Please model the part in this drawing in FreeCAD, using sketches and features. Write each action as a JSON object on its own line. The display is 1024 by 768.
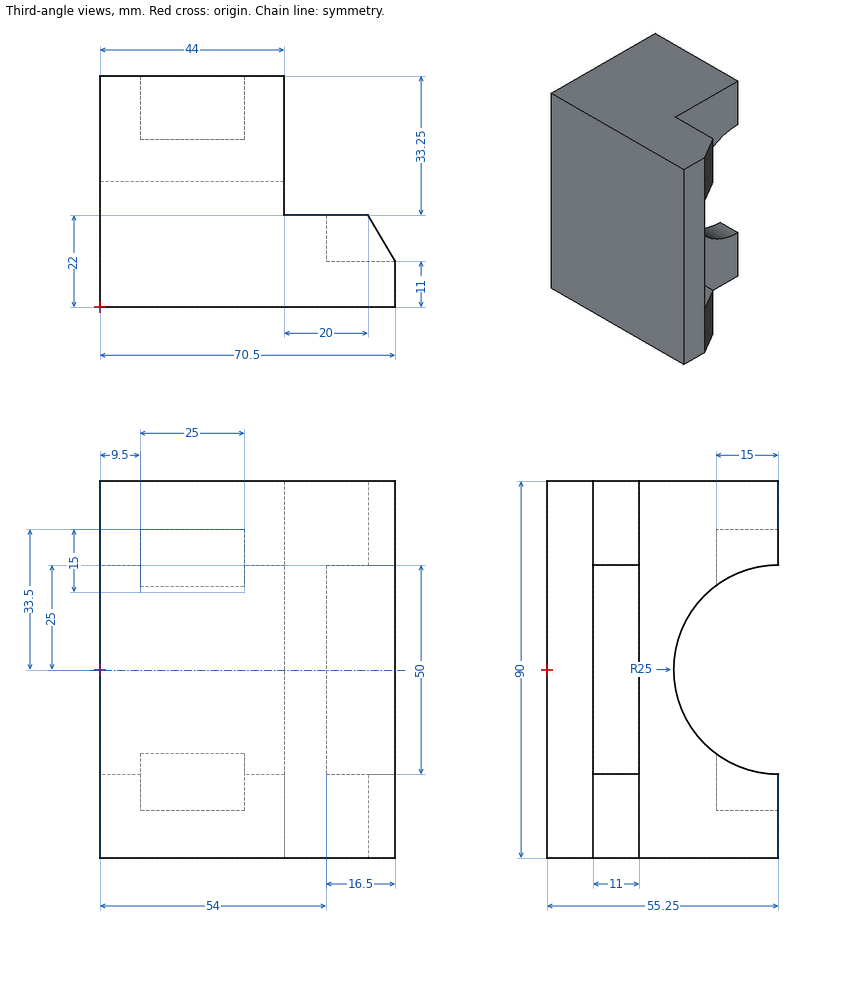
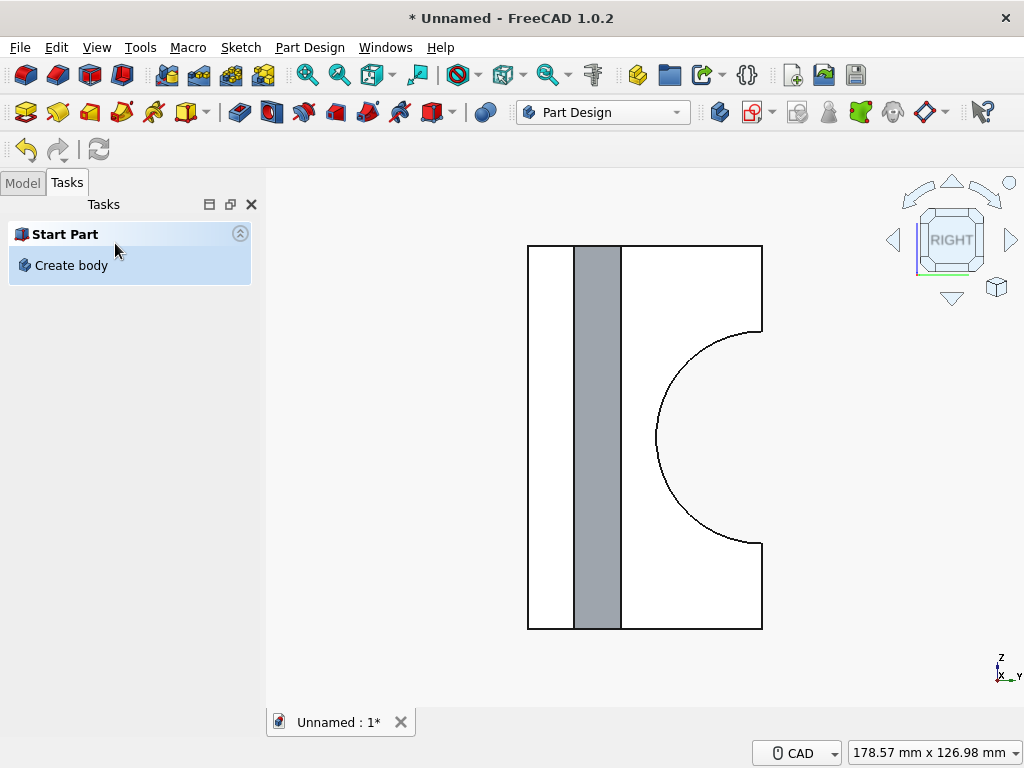
{"action": "key", "text": "4"}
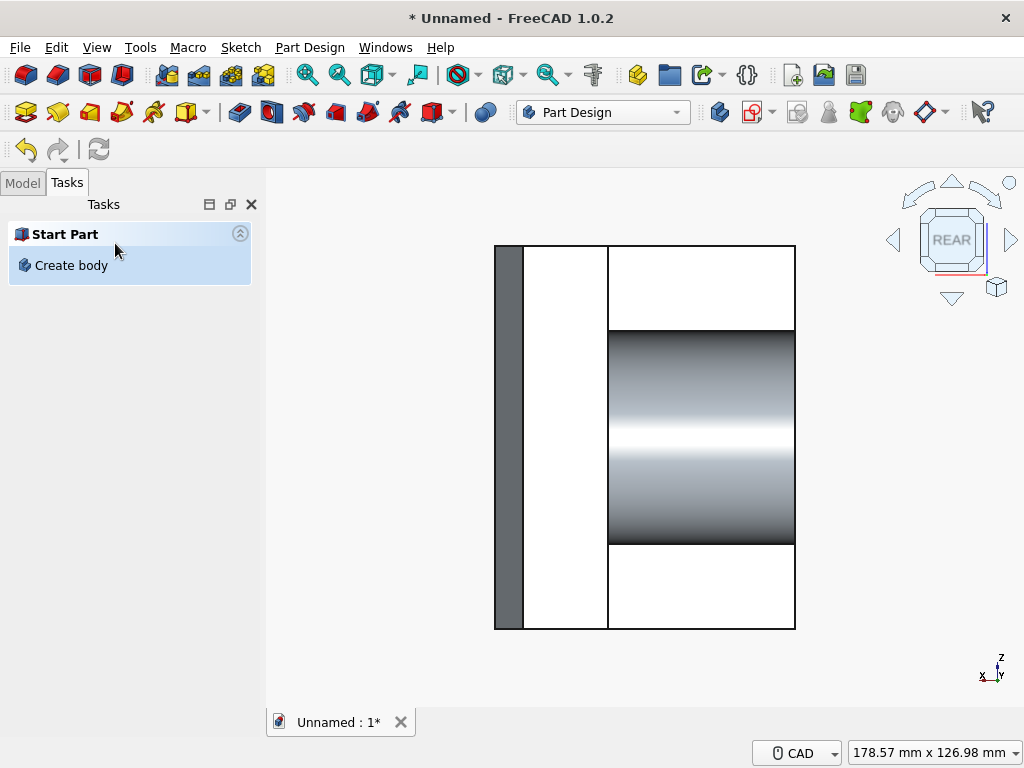
{"action": "left_click", "coordinate": [565, 327]}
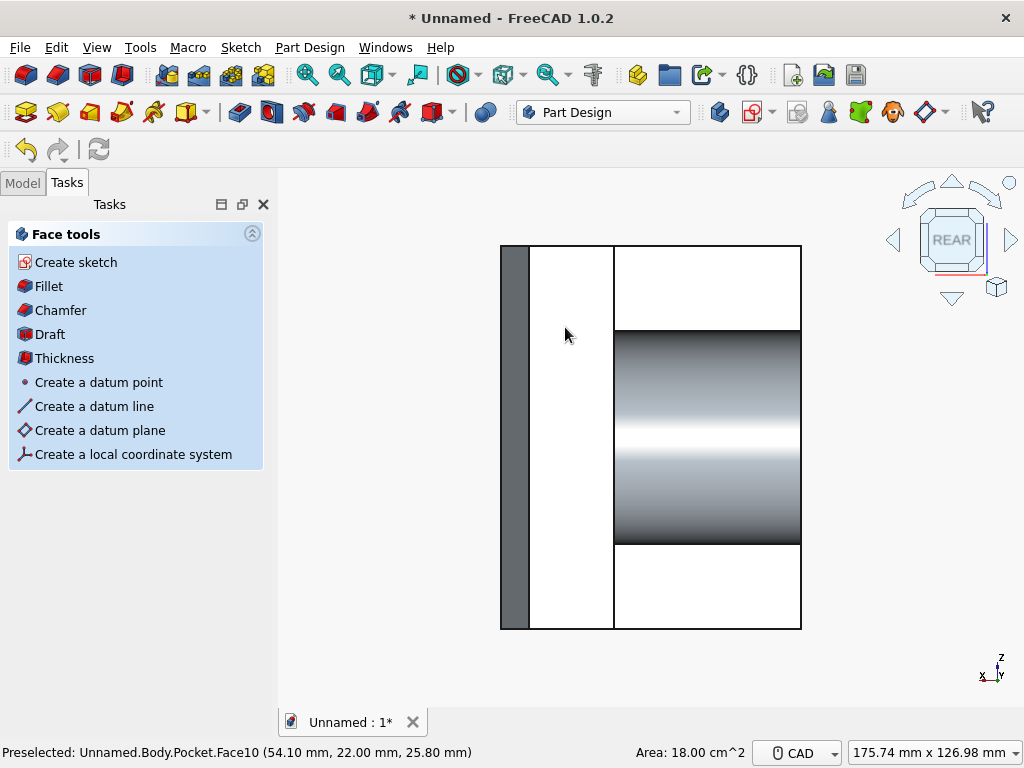
{"action": "left_click", "coordinate": [752, 112]}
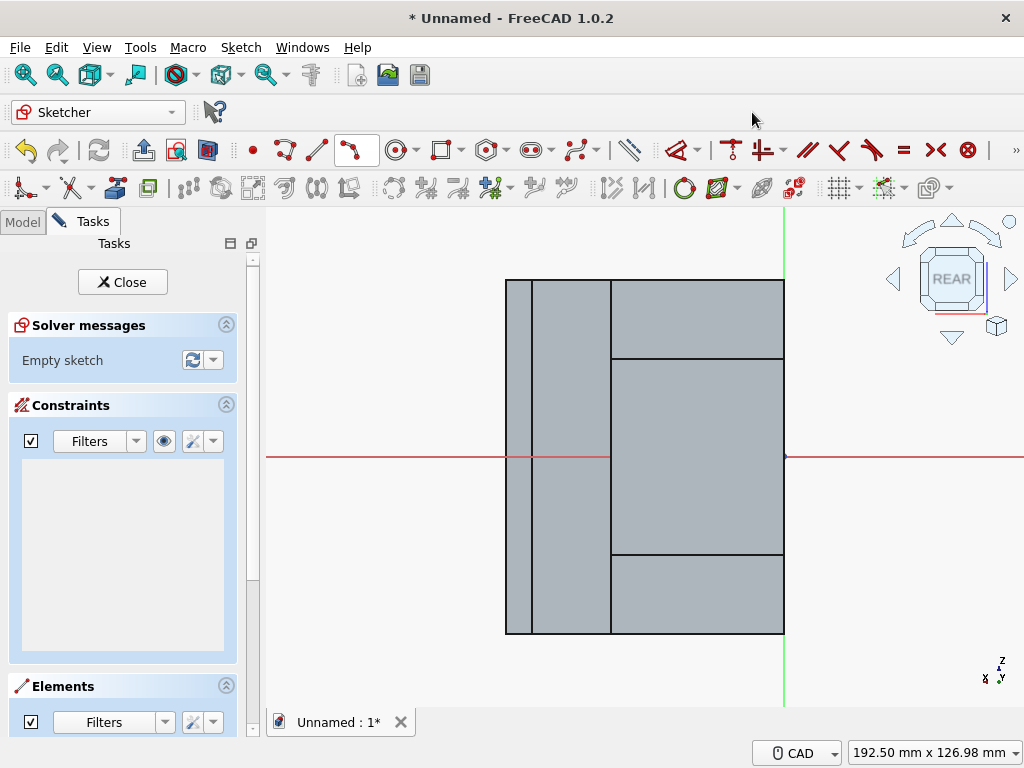
{"action": "left_click", "coordinate": [208, 150]}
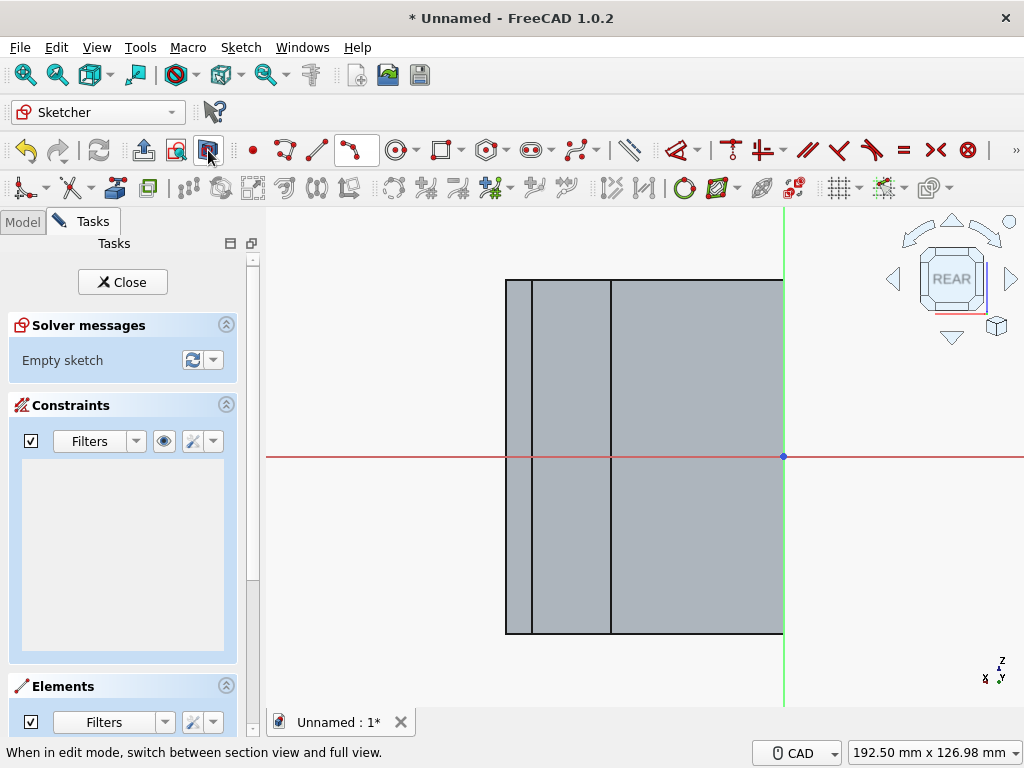
{"action": "scroll", "coordinate": [784, 457], "scroll_direction": "up", "scroll_amount": 2}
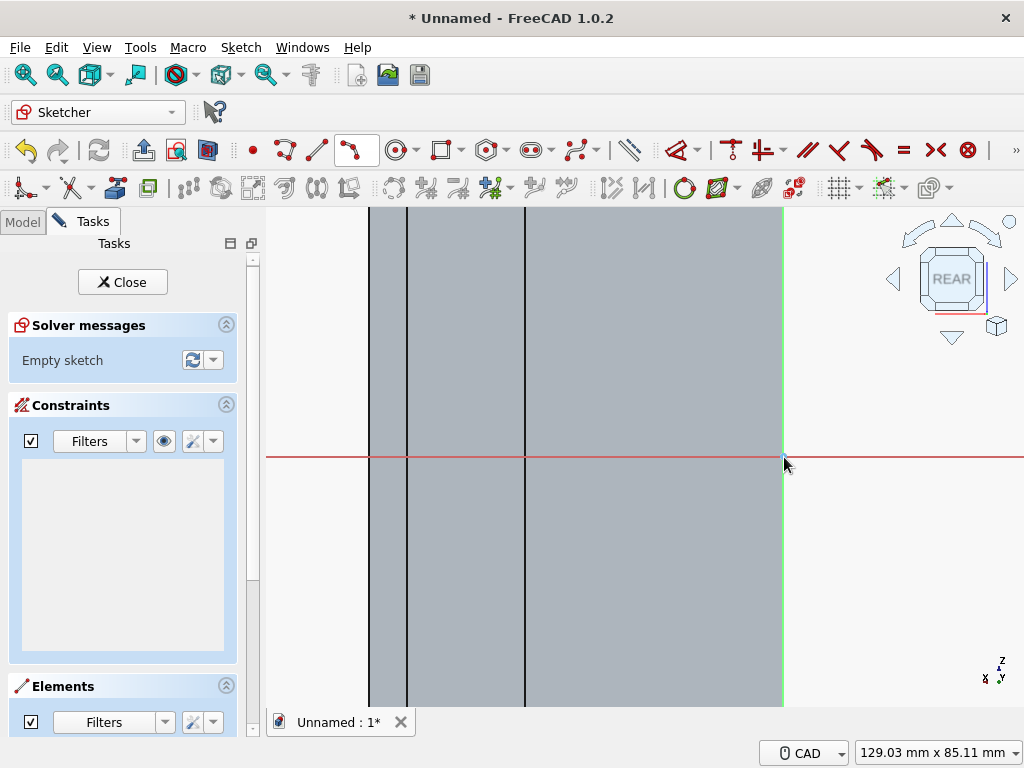
{"action": "left_click", "coordinate": [442, 150]}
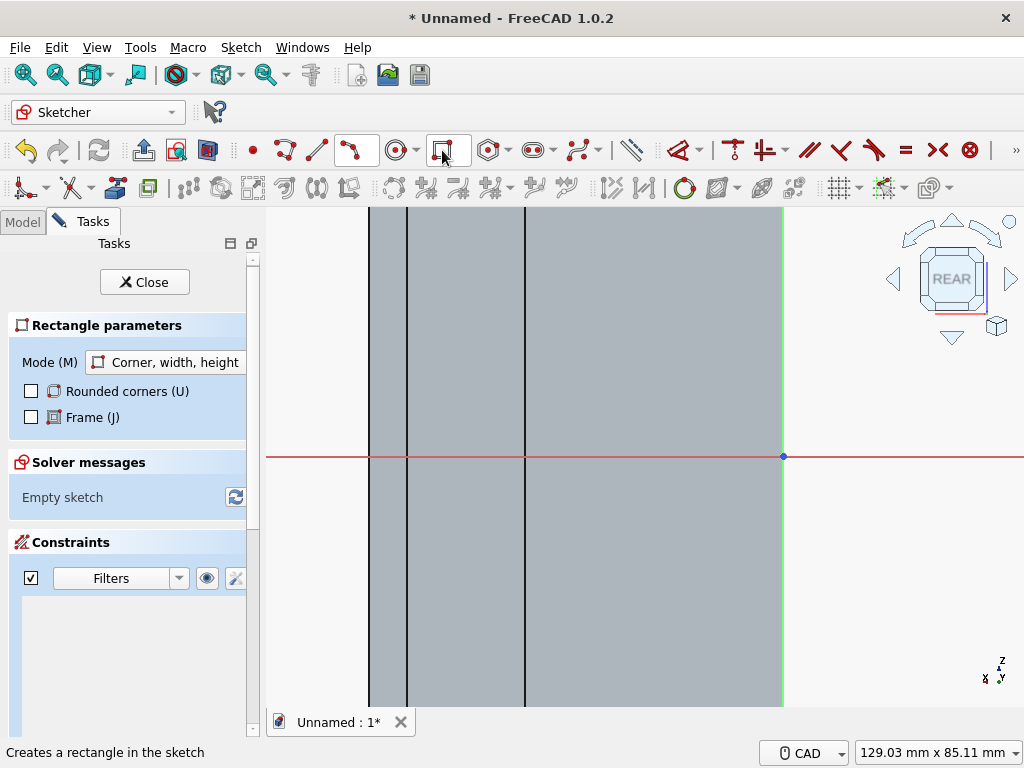
{"action": "left_click", "coordinate": [369, 310]}
{"action": "left_click", "coordinate": [466, 604]}
{"action": "key", "text": "Escape"}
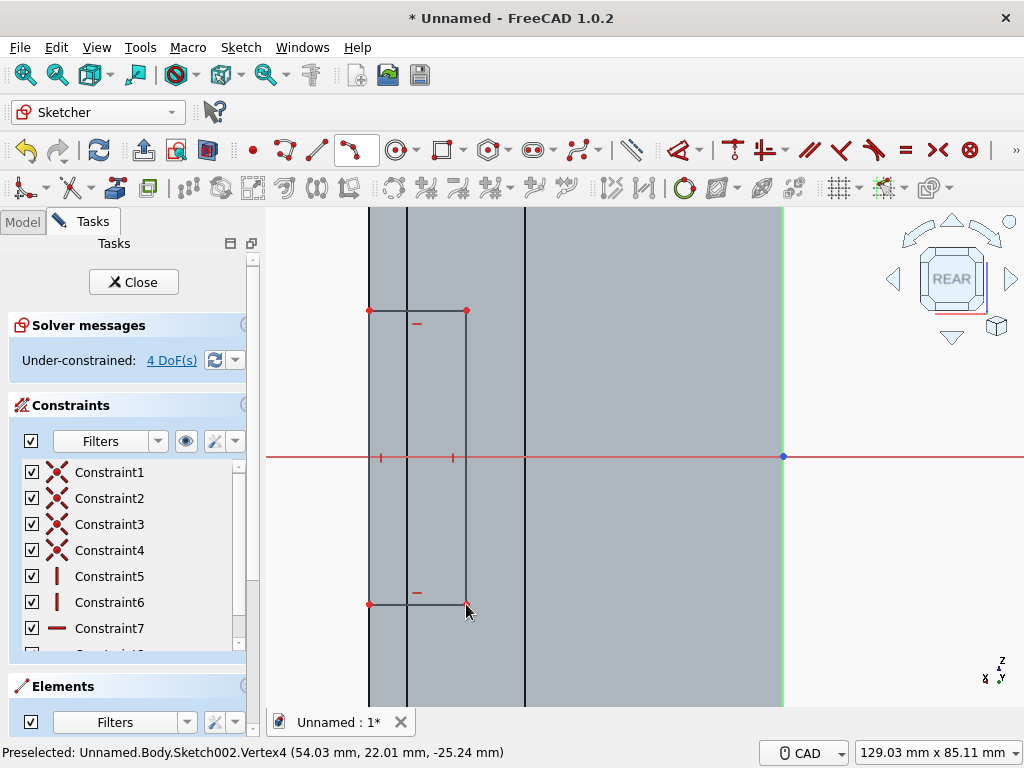
{"action": "left_click", "coordinate": [678, 150]}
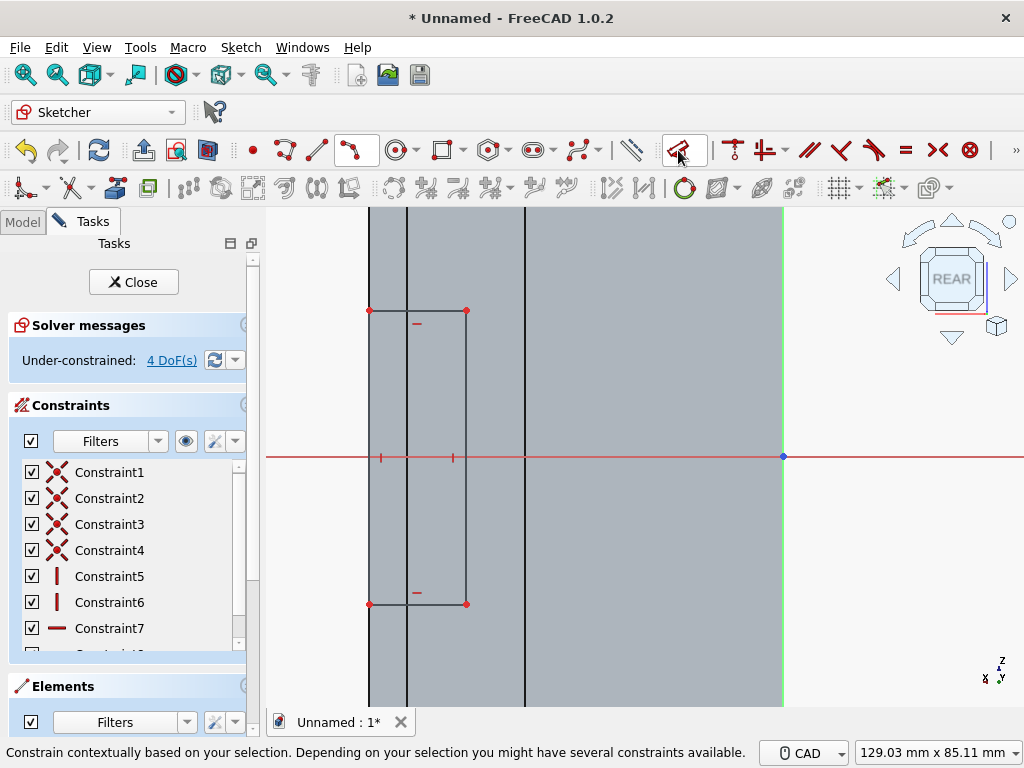
{"action": "left_click", "coordinate": [369, 399]}
{"action": "left_click", "coordinate": [335, 390]}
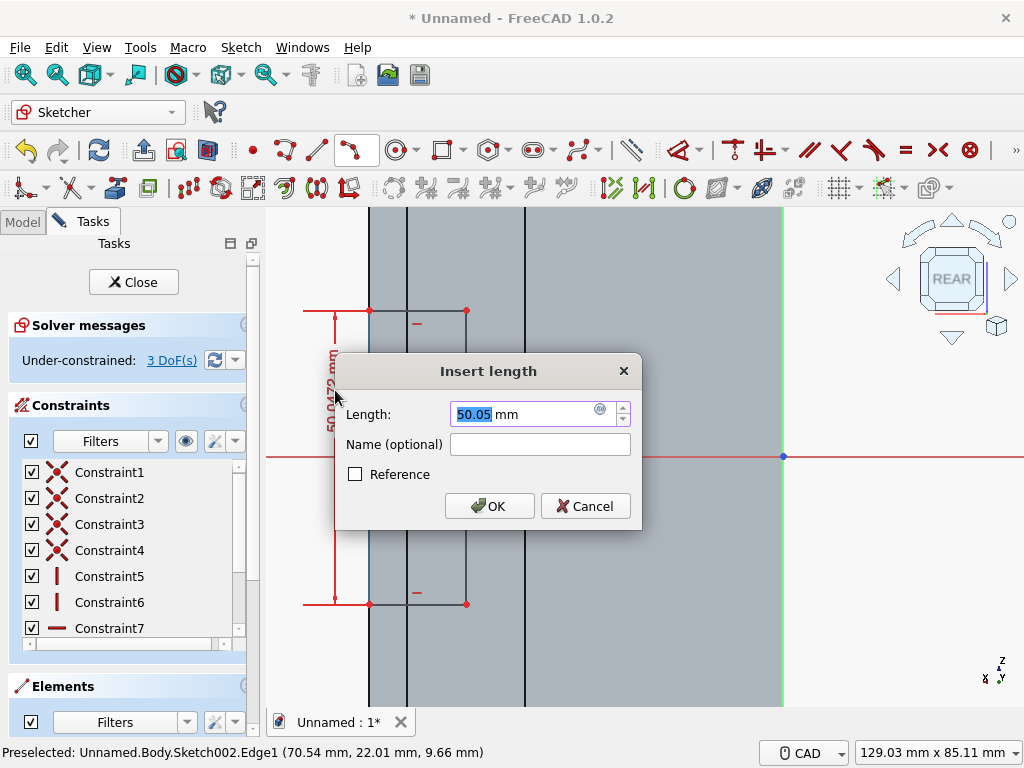
{"action": "type", "text": "50"}
{"action": "key", "text": "Return"}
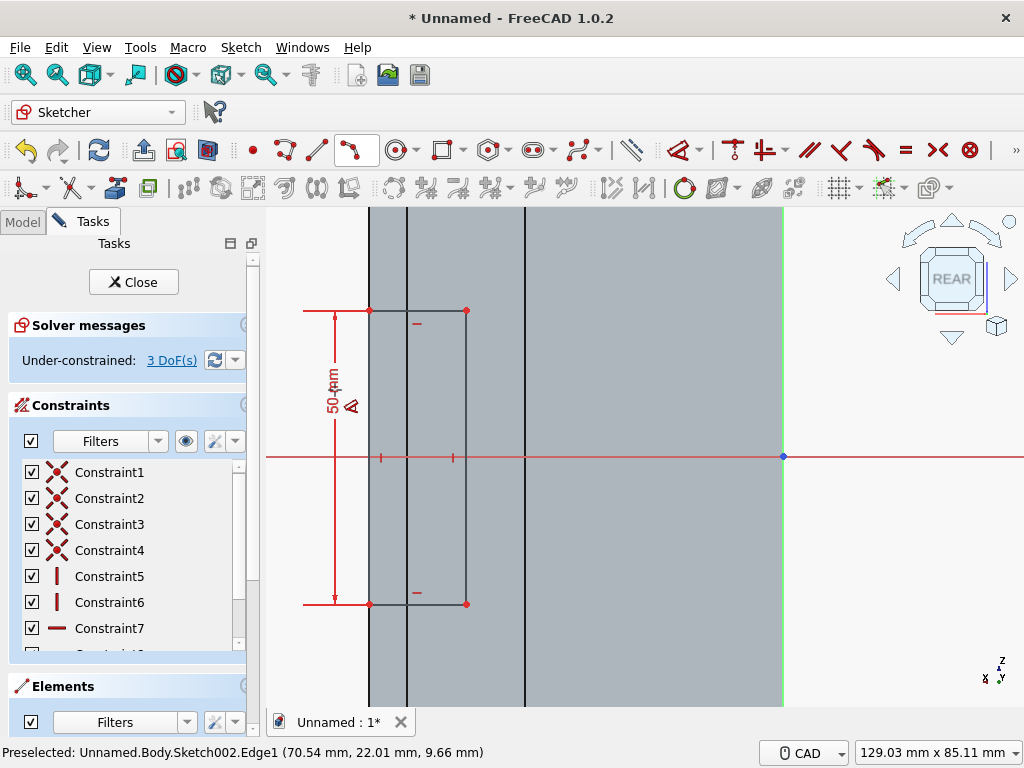
{"action": "left_click", "coordinate": [369, 311]}
{"action": "left_click", "coordinate": [335, 350]}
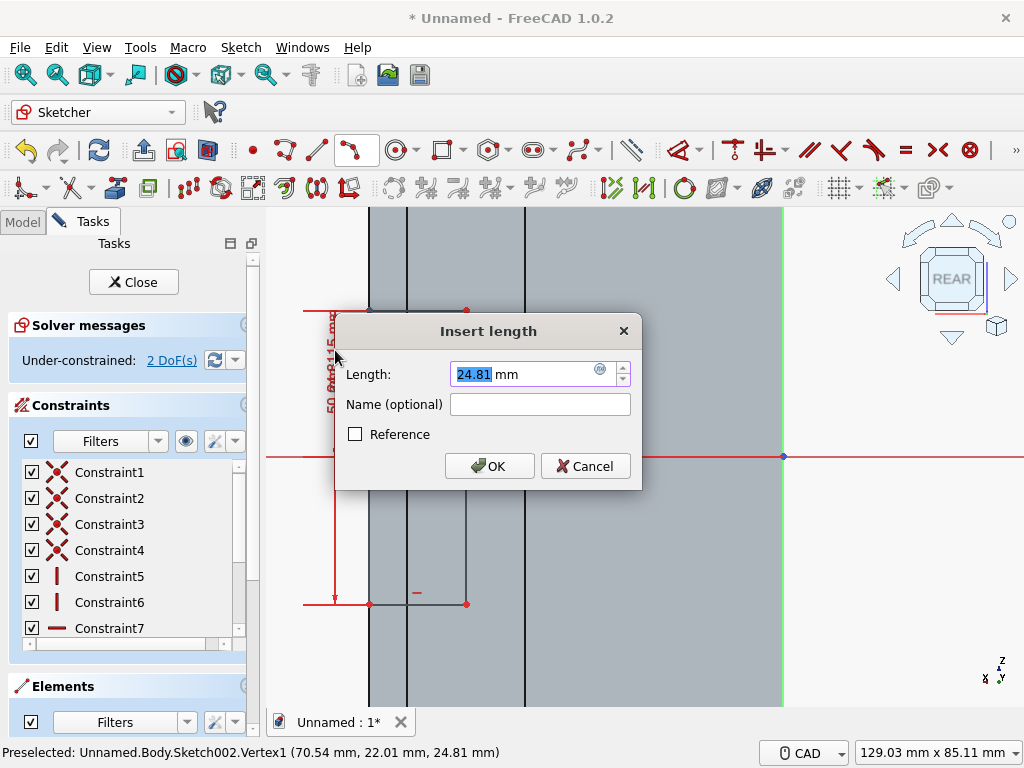
{"action": "type", "text": "25"}
{"action": "key", "text": "Return"}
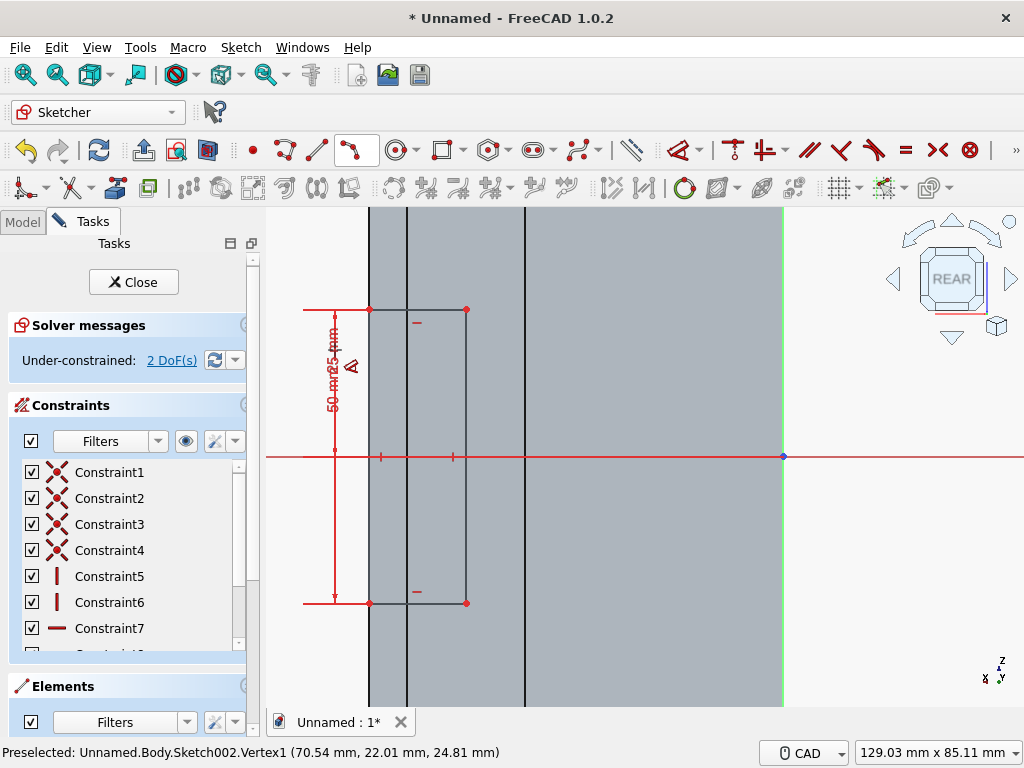
{"action": "left_click", "coordinate": [466, 604]}
{"action": "left_click", "coordinate": [625, 638]}